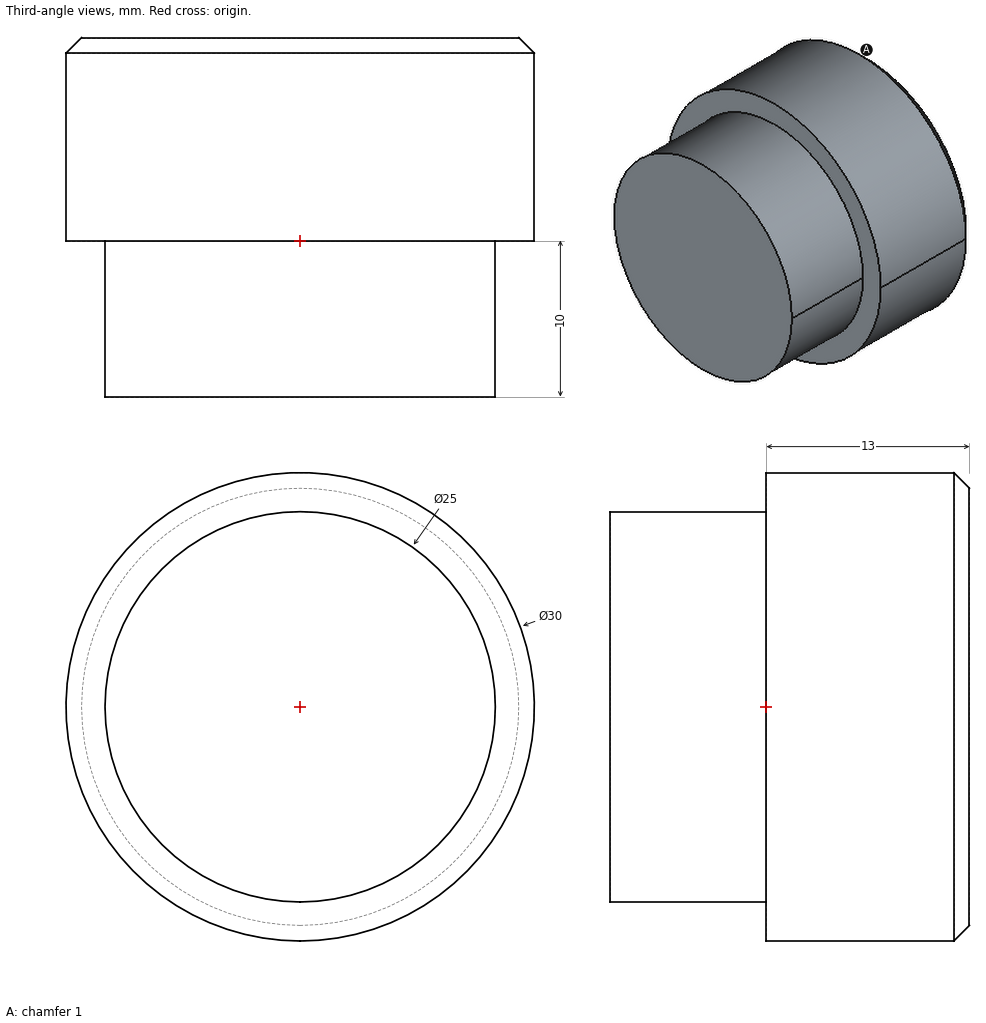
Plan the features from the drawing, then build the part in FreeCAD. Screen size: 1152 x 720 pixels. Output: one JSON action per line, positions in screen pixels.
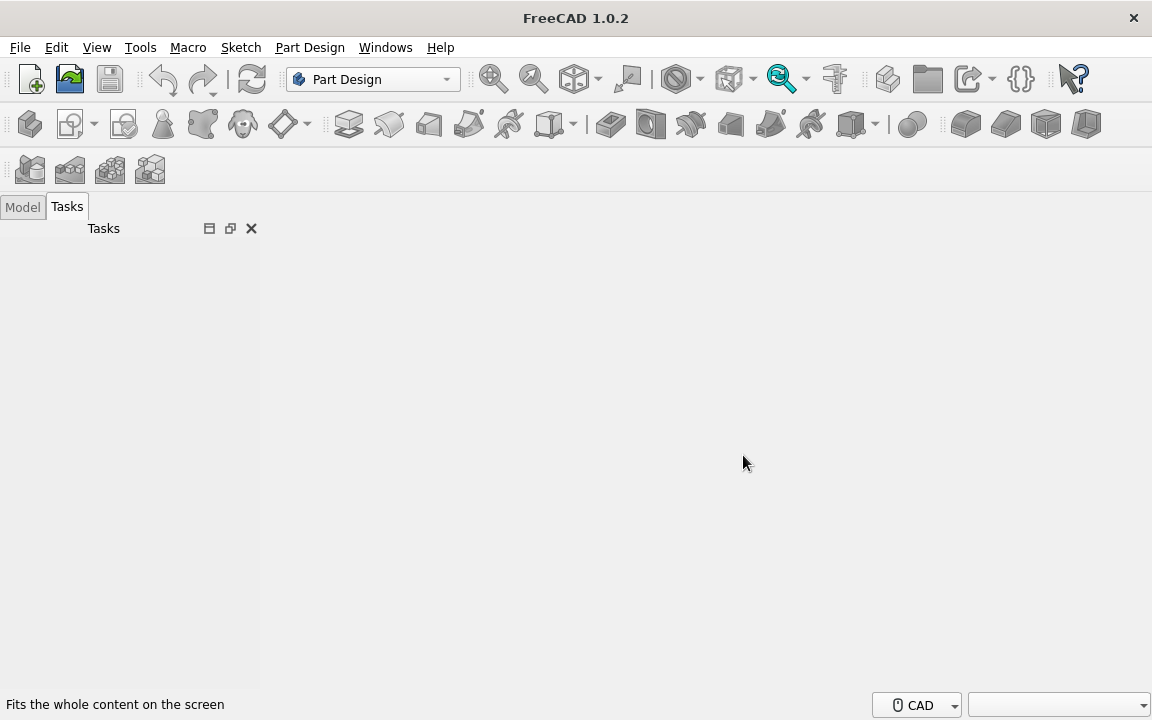
{"action": "left_click", "coordinate": [30, 80]}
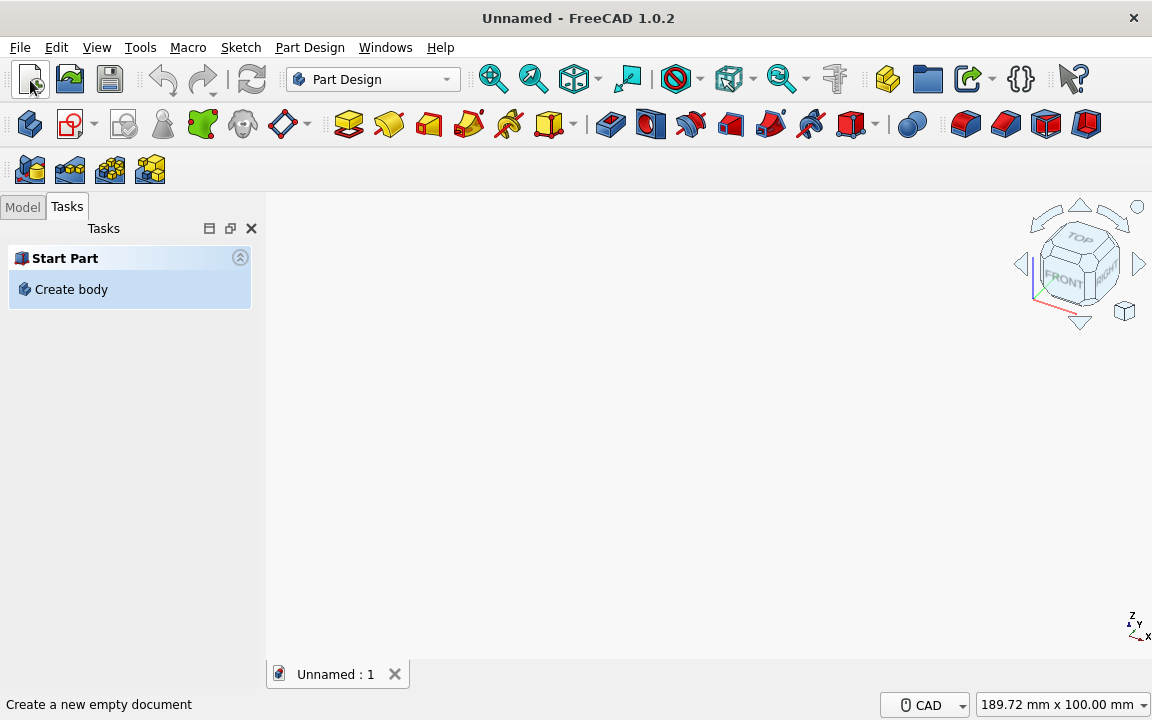
{"action": "left_click", "coordinate": [70, 124]}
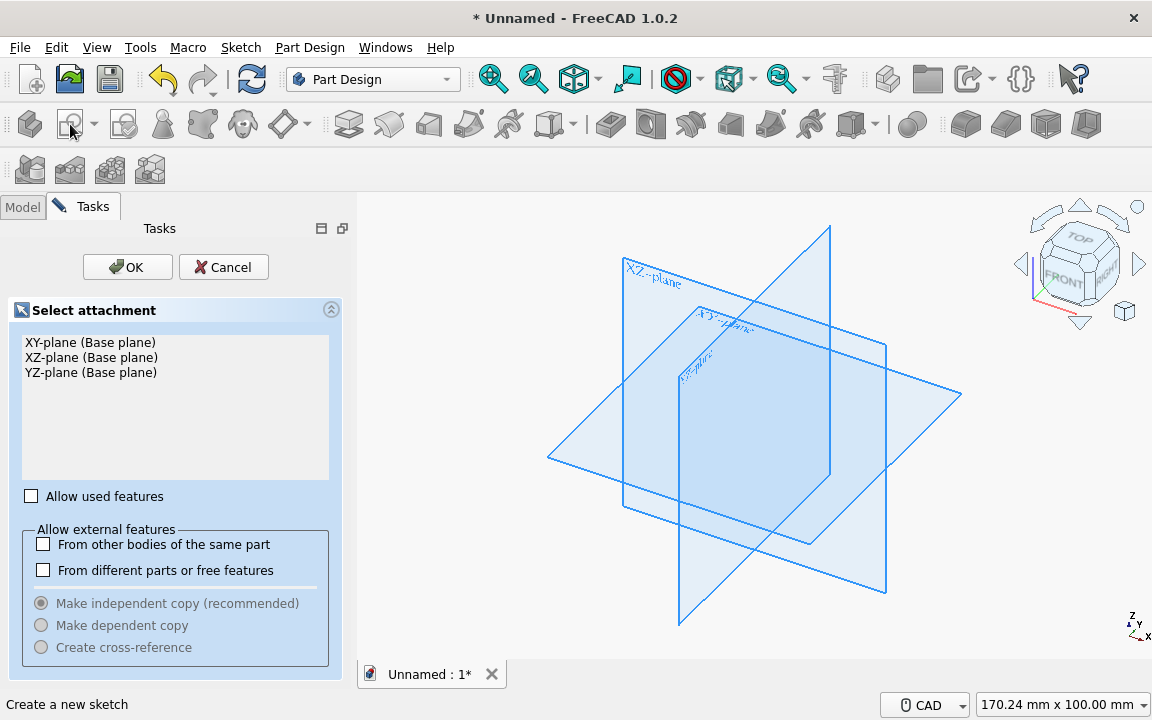
{"action": "left_click", "coordinate": [82, 358]}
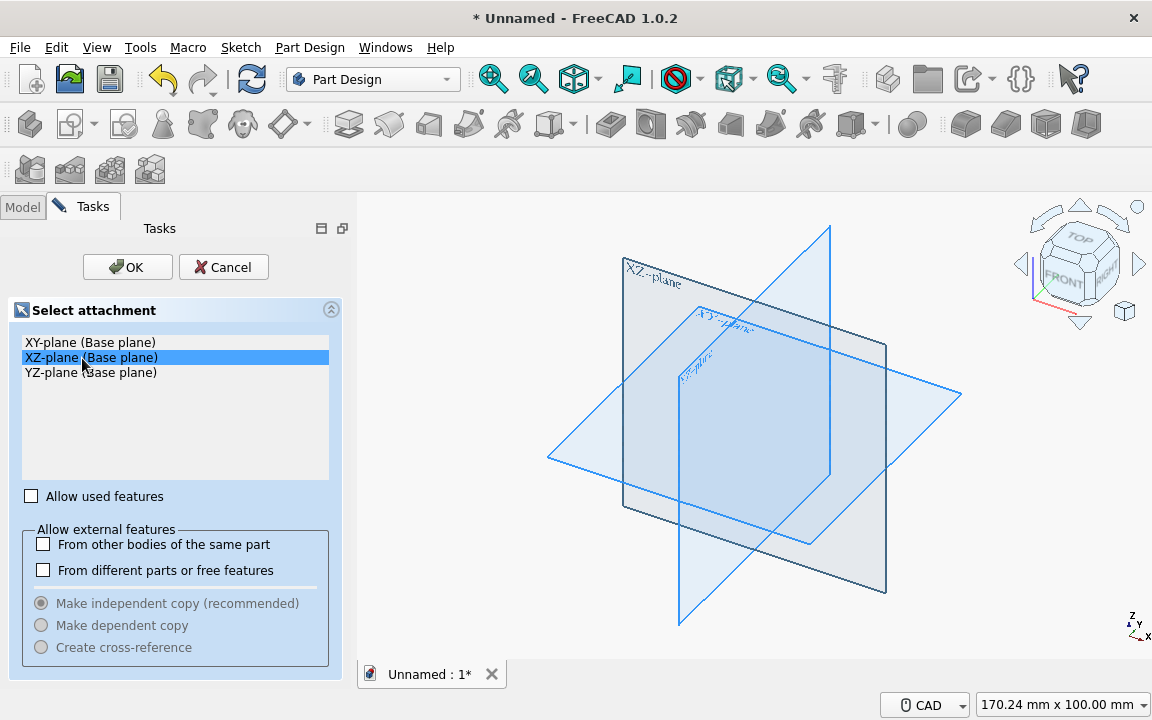
{"action": "left_click", "coordinate": [128, 267]}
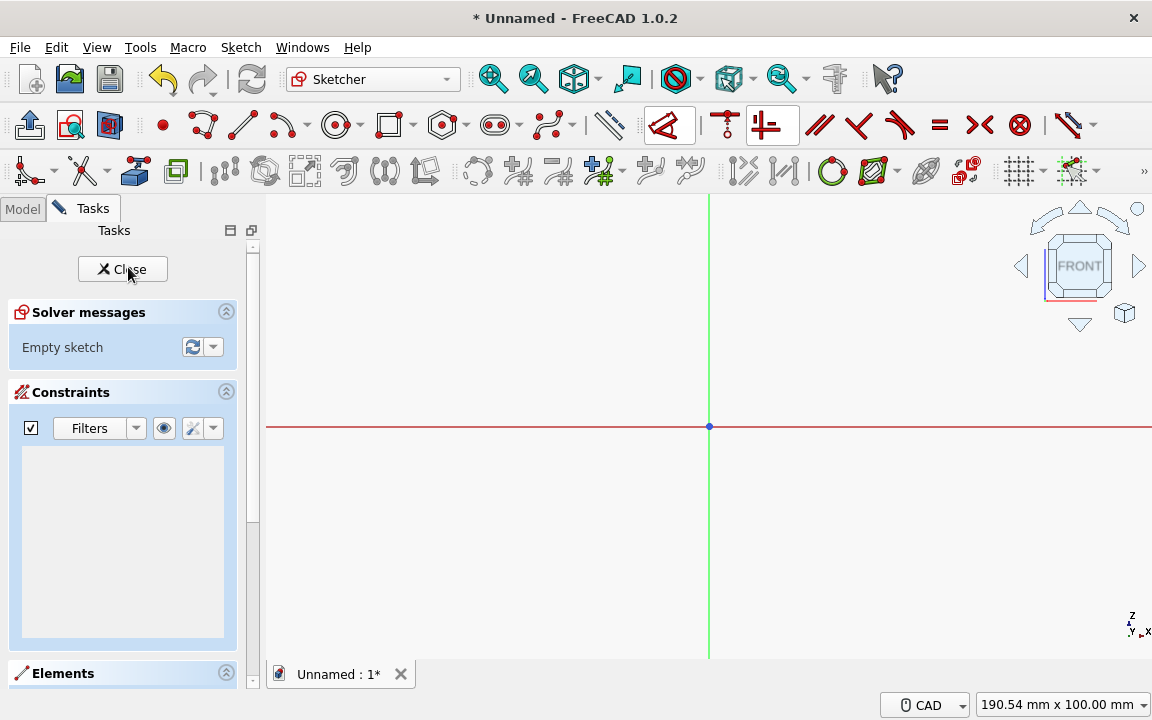
{"action": "scroll", "coordinate": [765, 426], "scroll_direction": "up", "scroll_amount": 4}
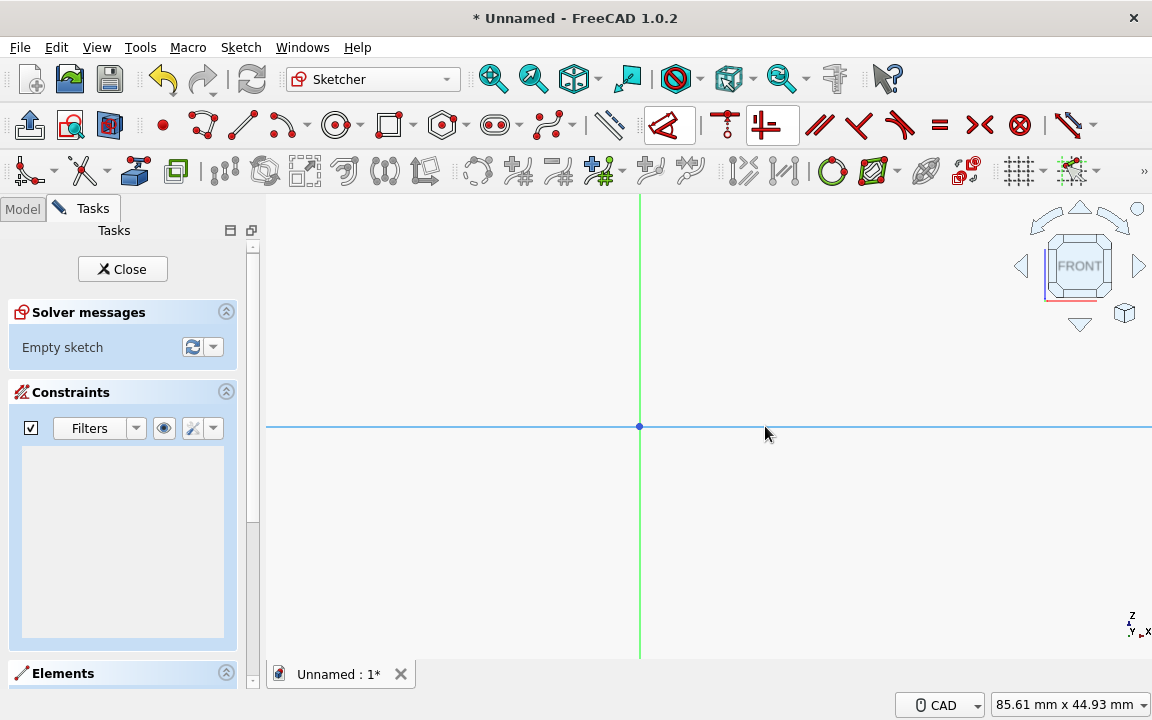
{"action": "left_click", "coordinate": [336, 126]}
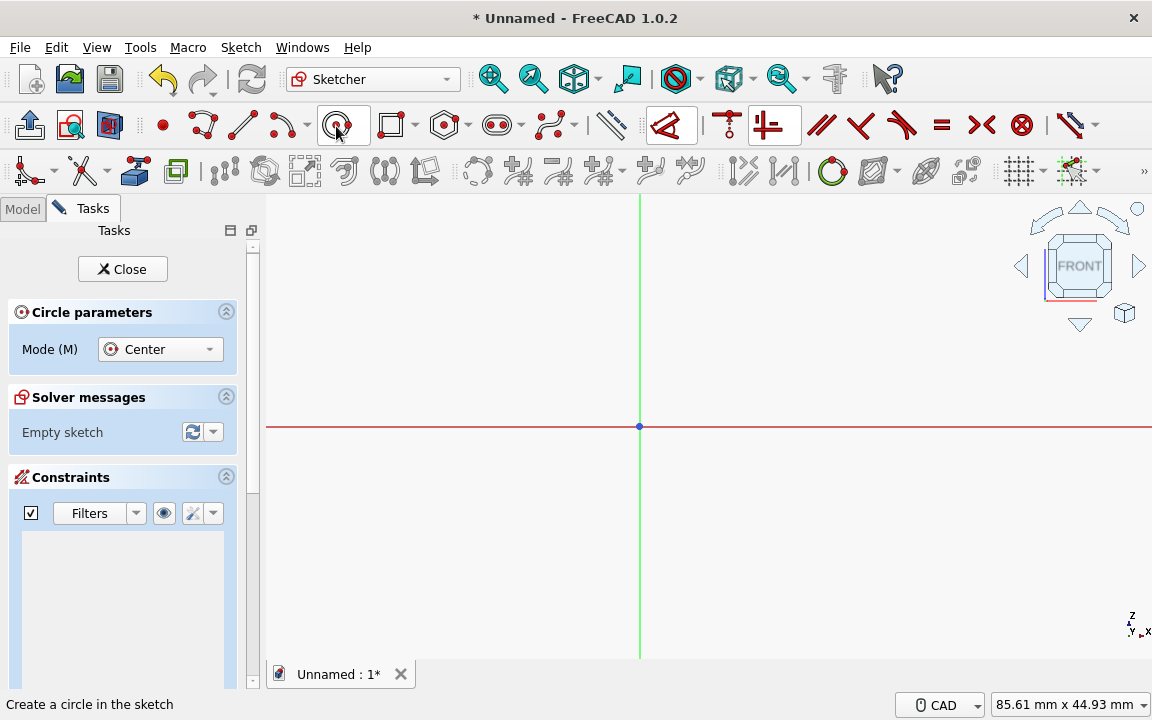
{"action": "left_click", "coordinate": [640, 426]}
{"action": "mouse_move", "coordinate": [749, 317]}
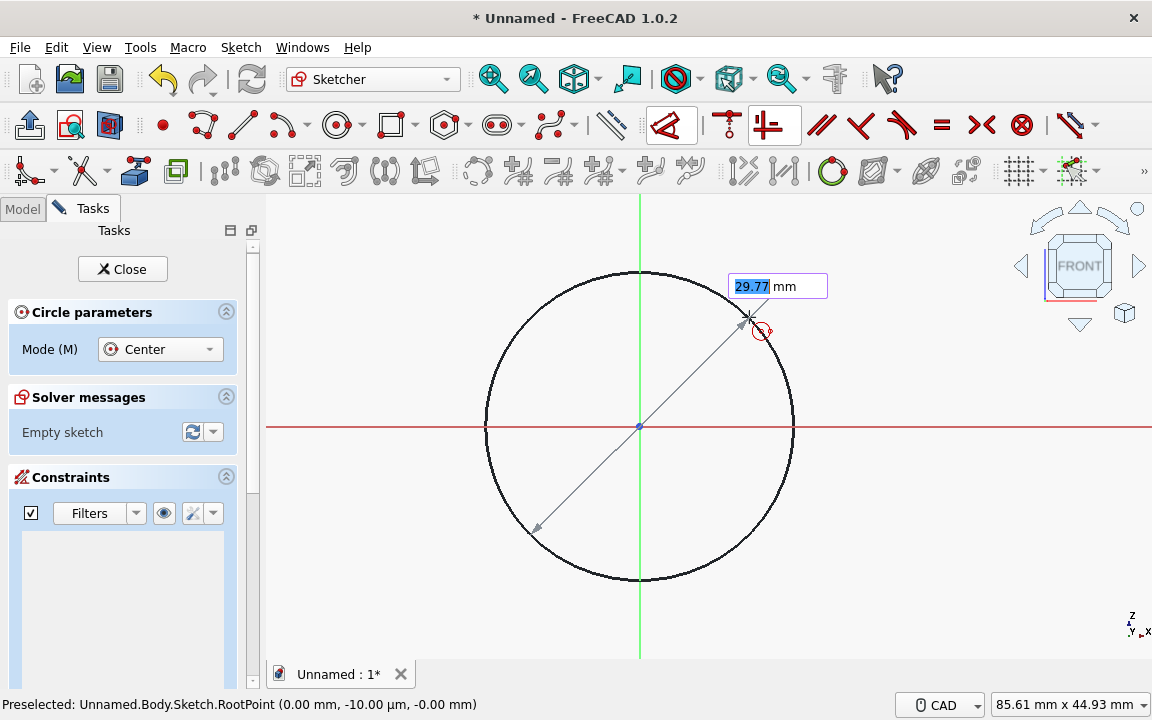
{"action": "type", "text": "30"}
{"action": "key", "text": "Return"}
{"action": "key", "text": "Escape"}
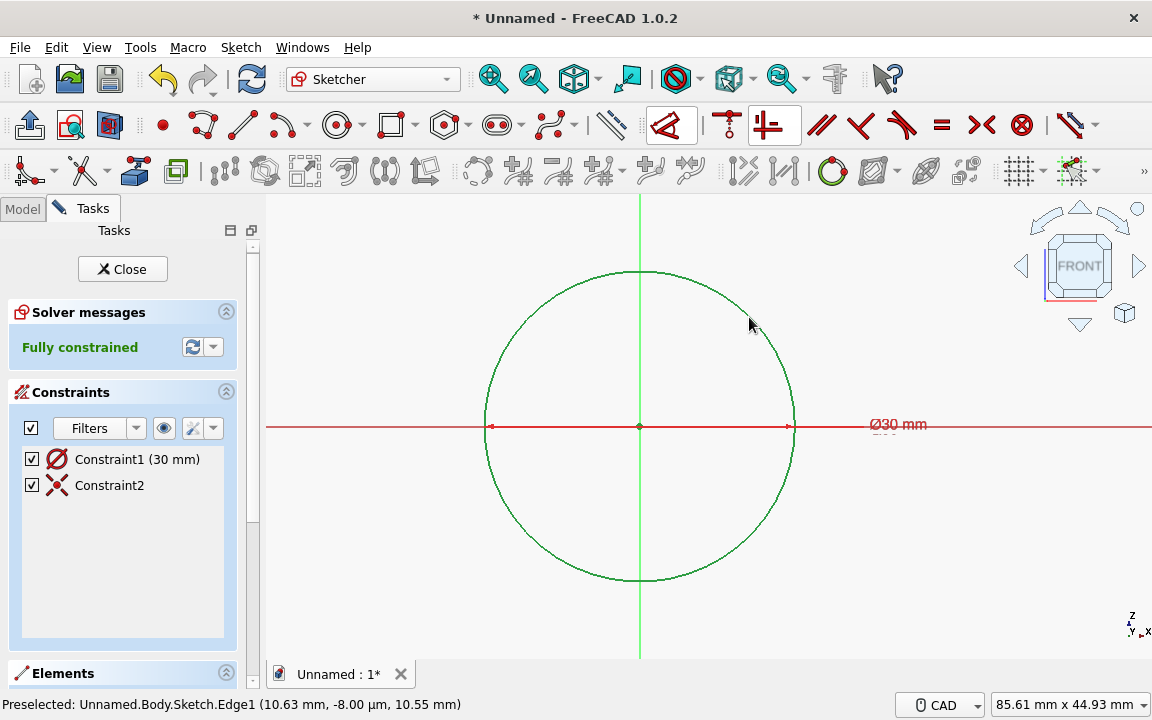
{"action": "left_click", "coordinate": [123, 269]}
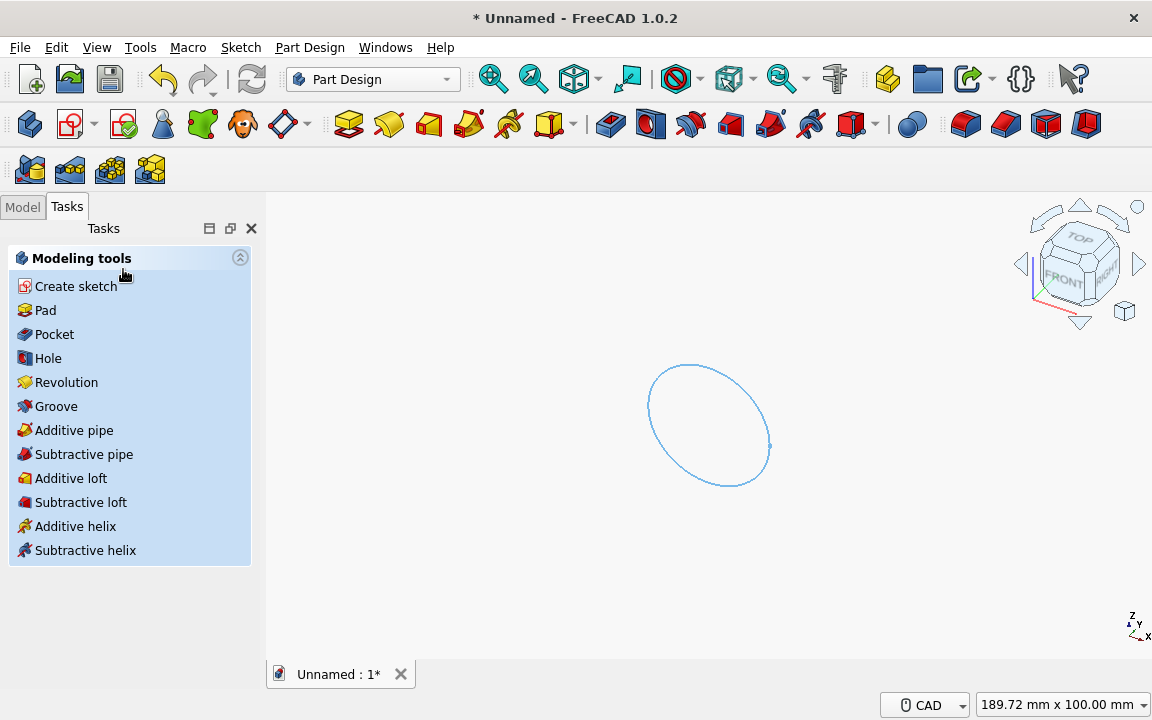
{"action": "left_click", "coordinate": [350, 124]}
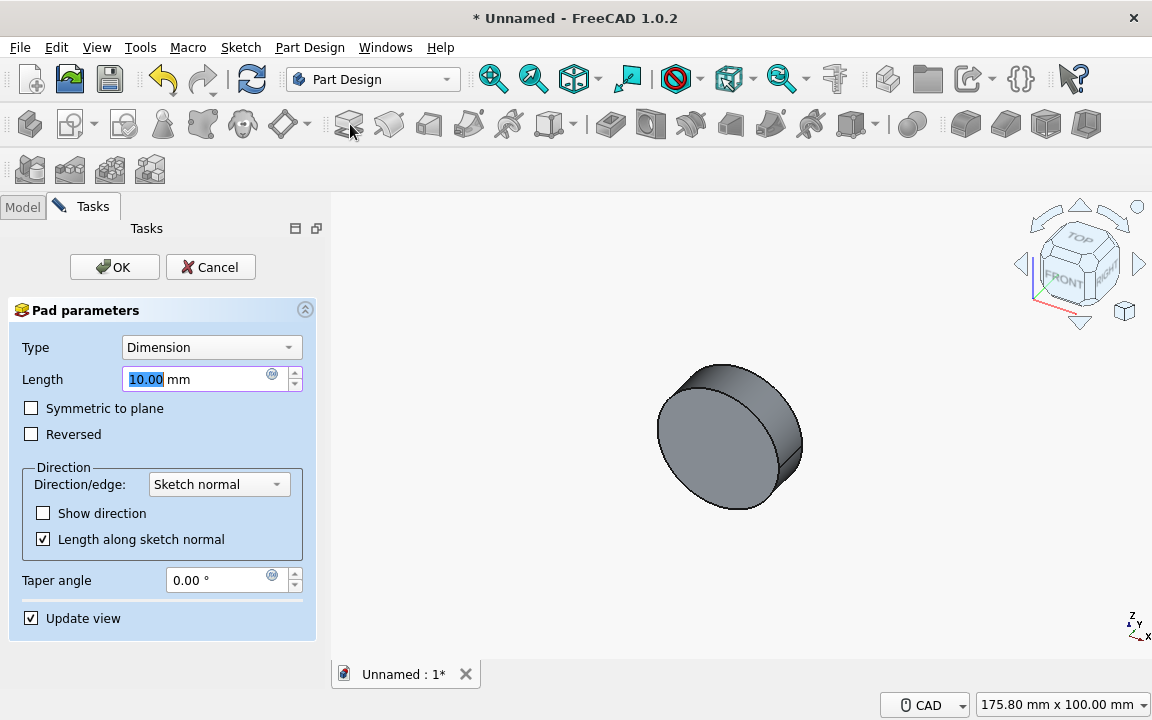
{"action": "type", "text": "13"}
{"action": "key", "text": "Tab"}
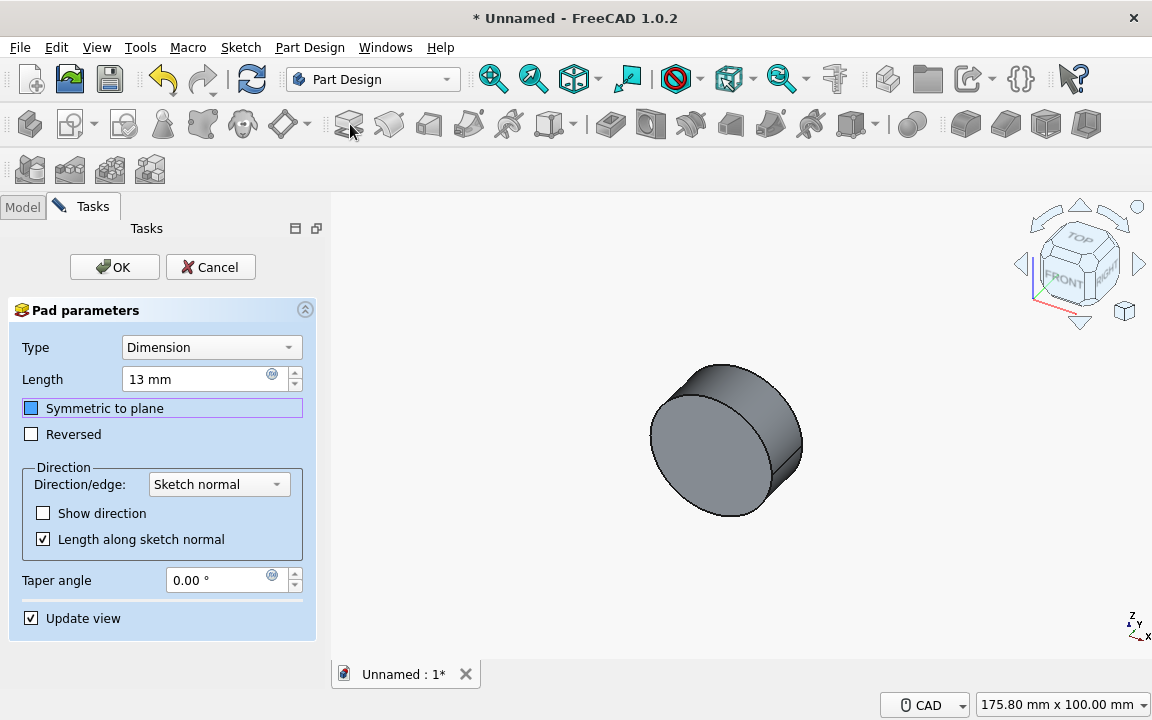
{"action": "left_click", "coordinate": [30, 434]}